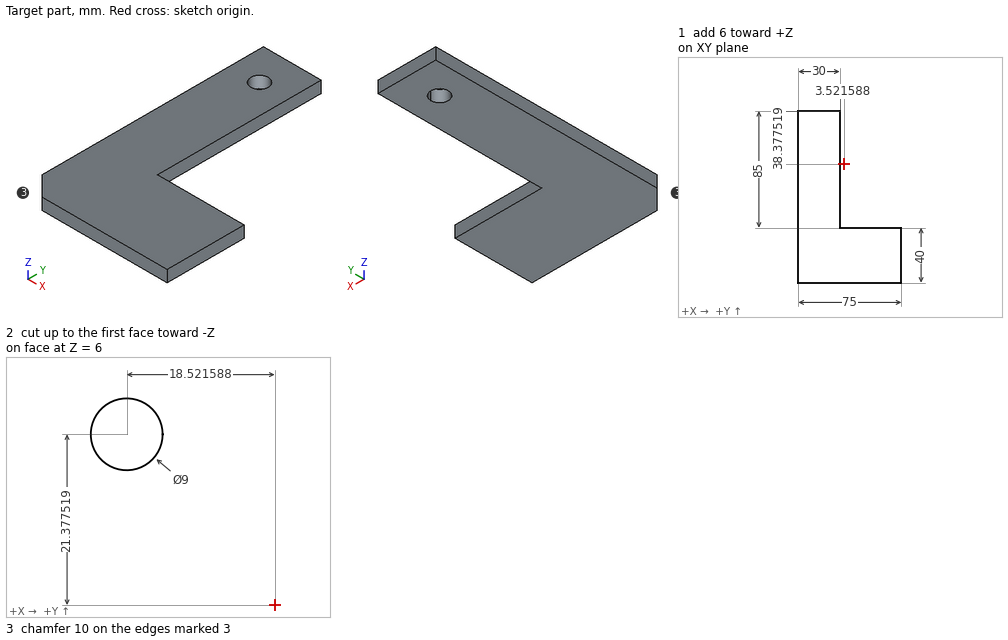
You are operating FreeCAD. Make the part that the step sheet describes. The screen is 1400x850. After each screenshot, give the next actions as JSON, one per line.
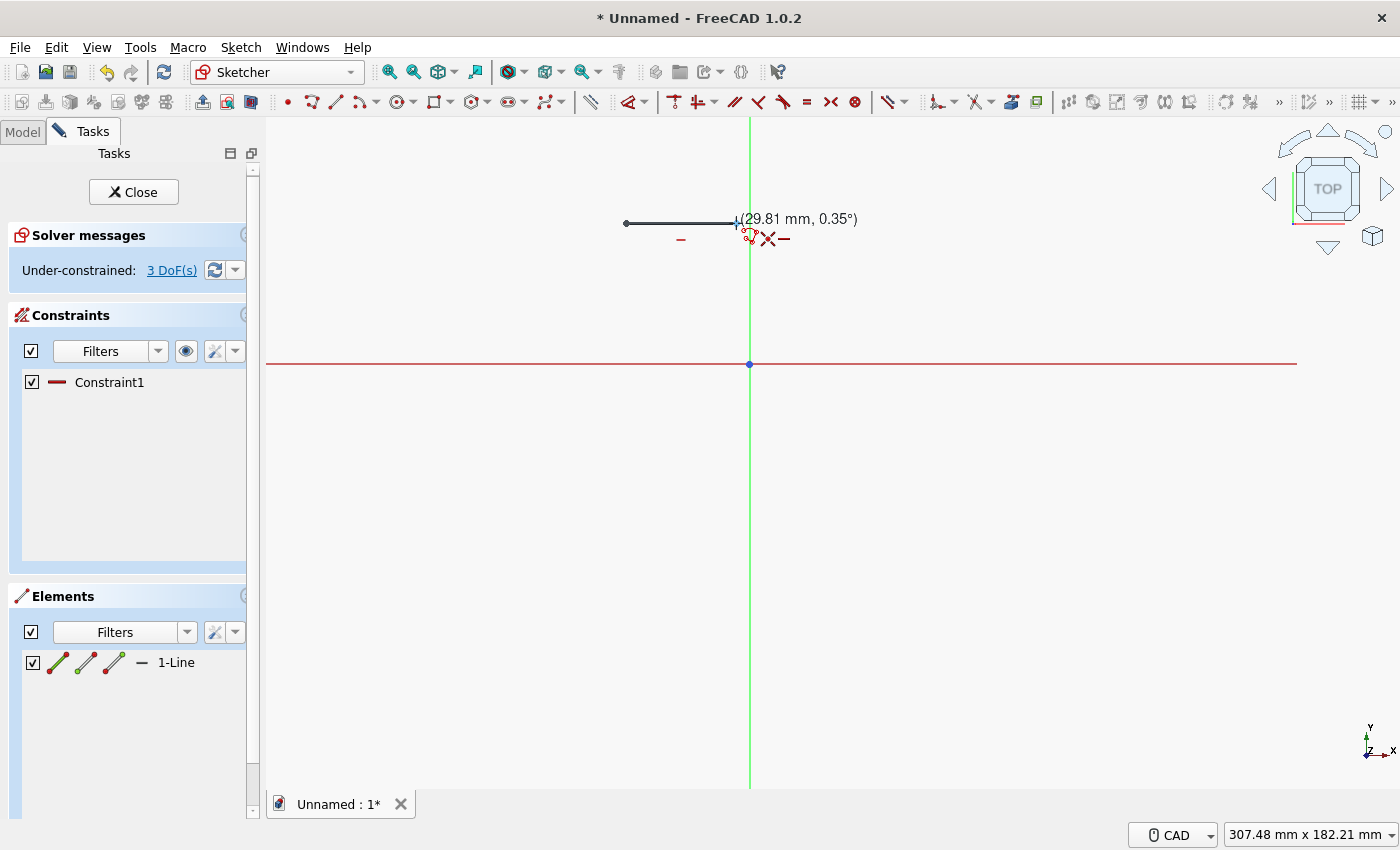
{"action": "left_click", "coordinate": [626, 684]}
{"action": "left_click", "coordinate": [903, 684]}
{"action": "left_click", "coordinate": [903, 536]}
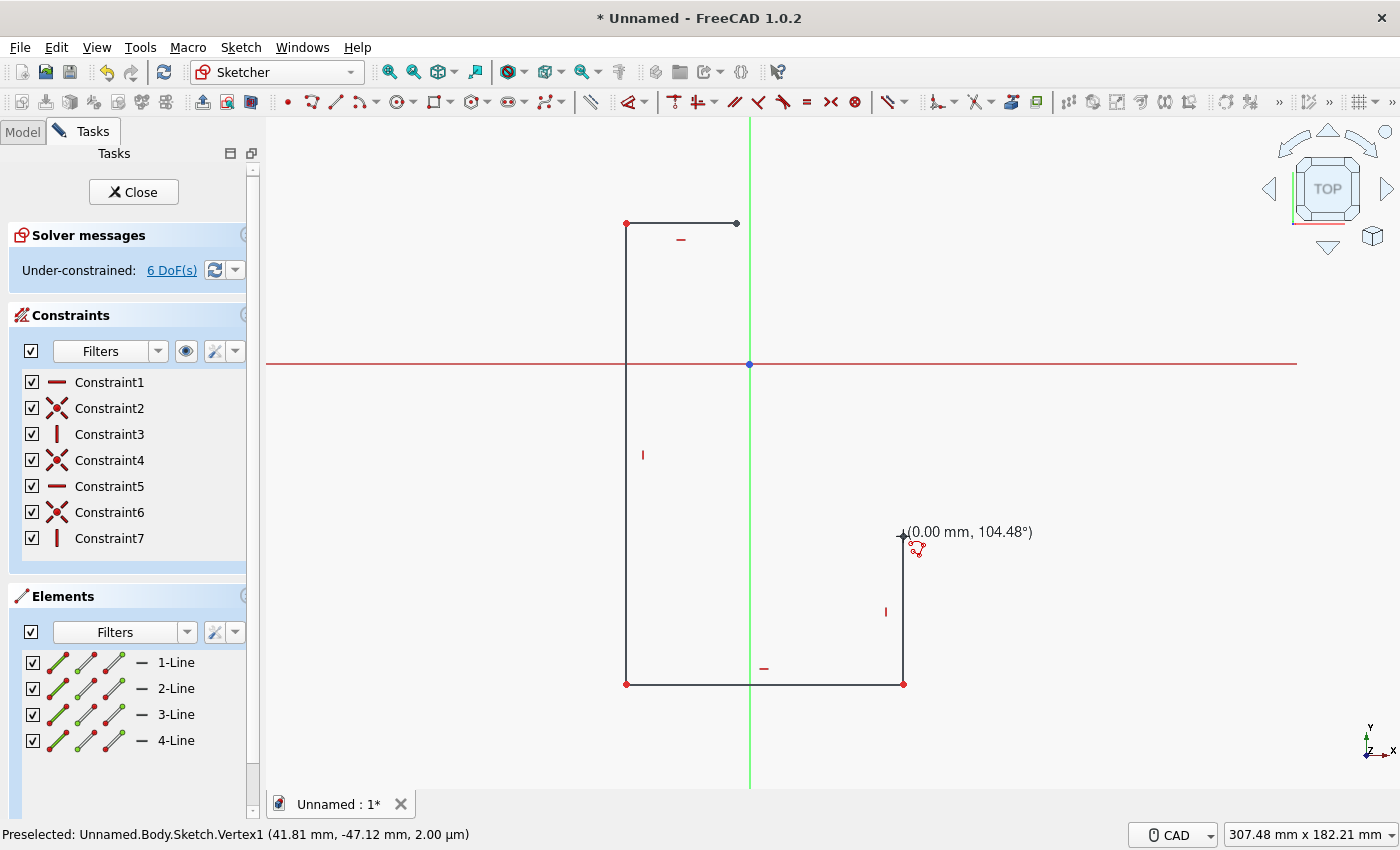
{"action": "scroll", "coordinate": [737, 536], "scroll_direction": "up", "scroll_amount": 2}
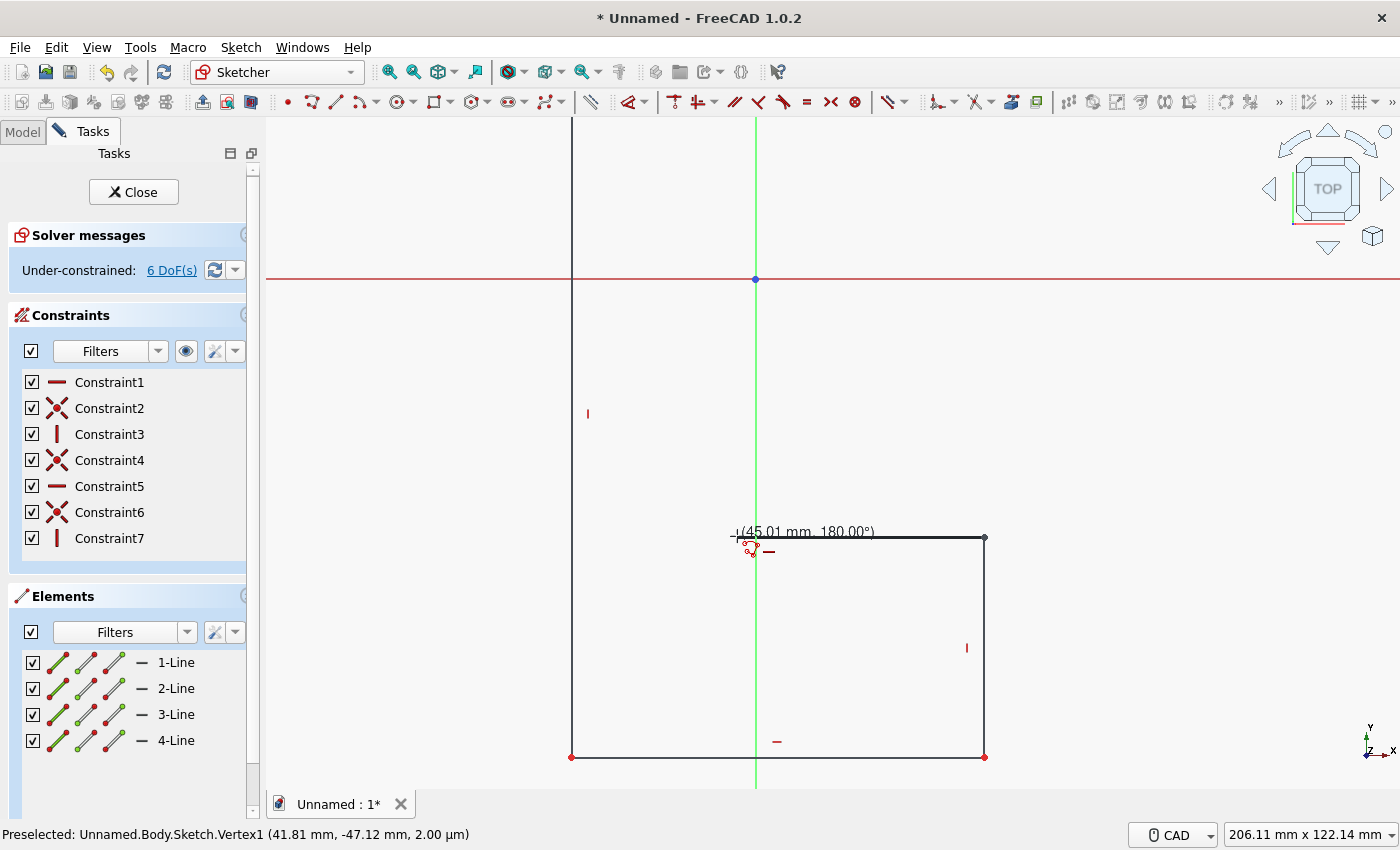
{"action": "left_click", "coordinate": [737, 536]}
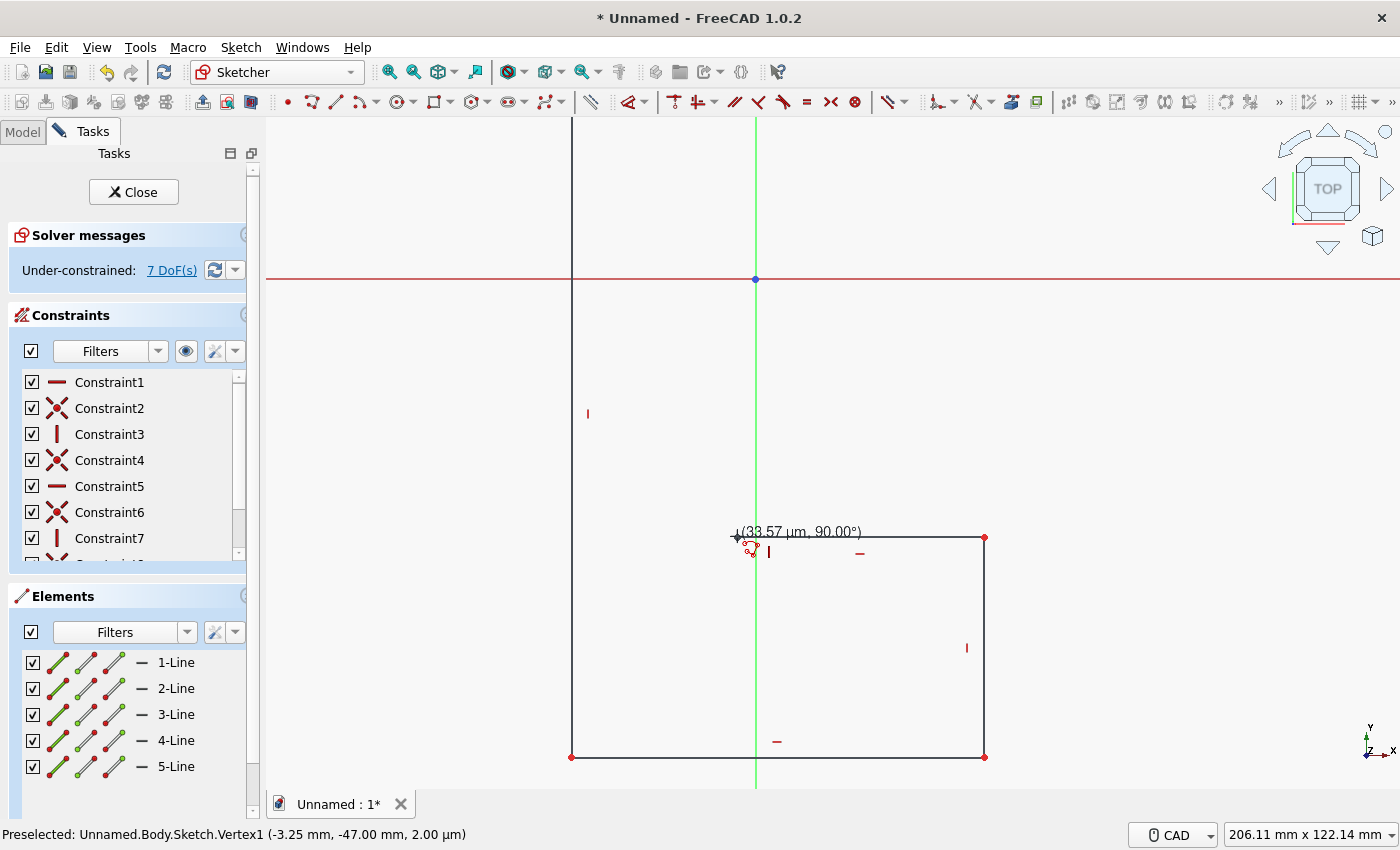
{"action": "scroll", "coordinate": [737, 536], "scroll_direction": "down", "scroll_amount": 2}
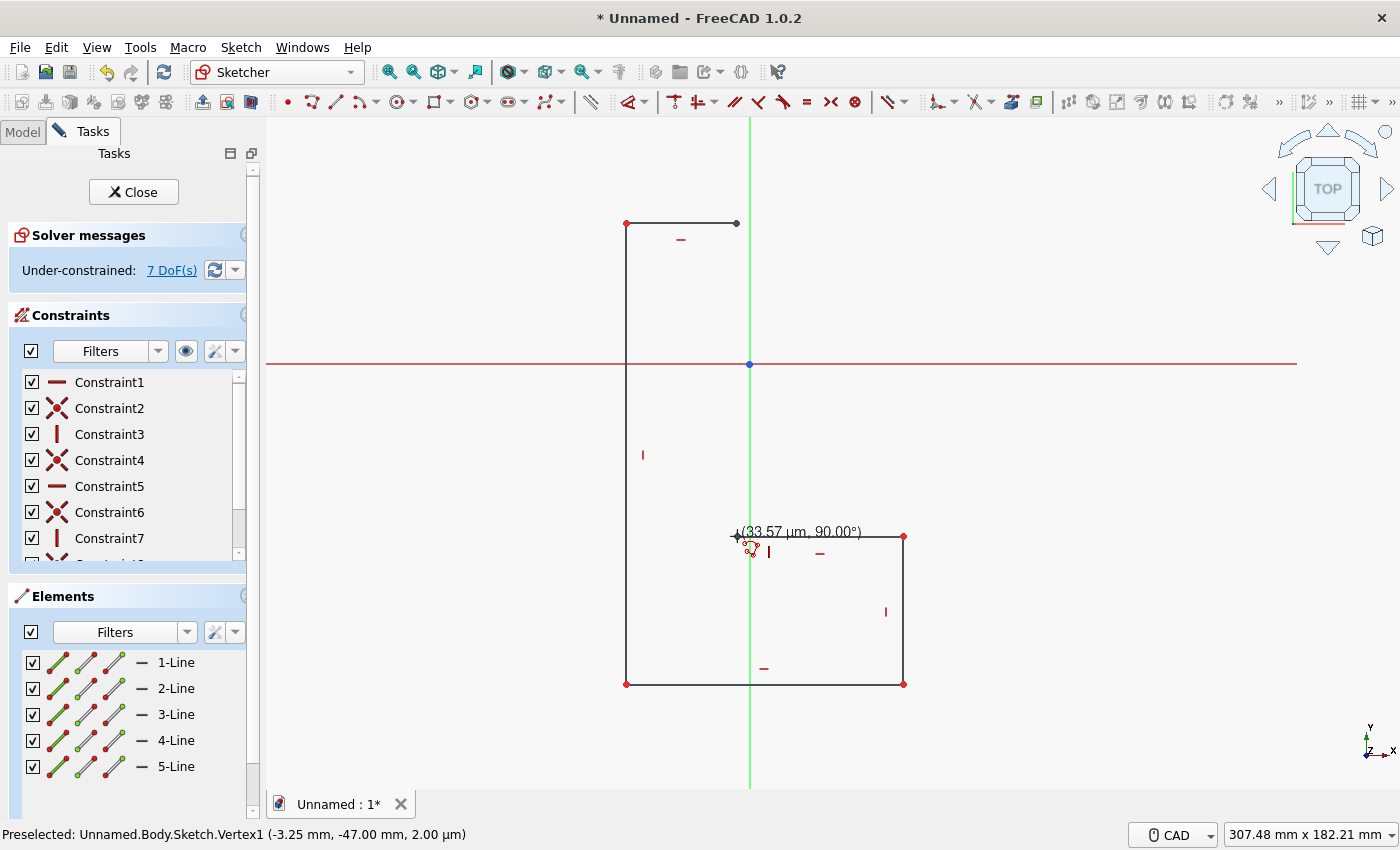
{"action": "scroll", "coordinate": [737, 223], "scroll_direction": "up", "scroll_amount": 2}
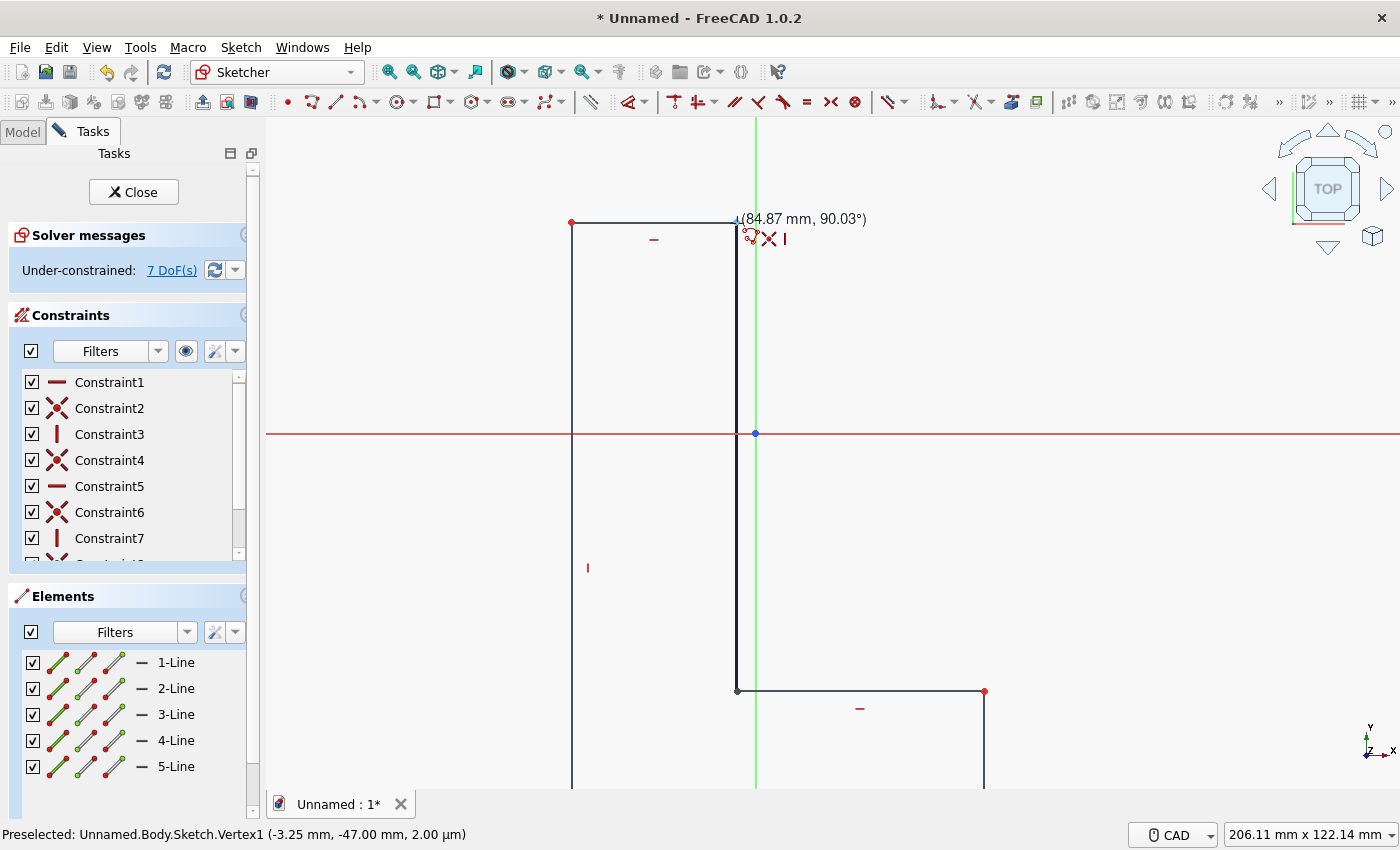
{"action": "left_click", "coordinate": [737, 223]}
{"action": "key", "text": "Escape"}
{"action": "key", "text": "Escape"}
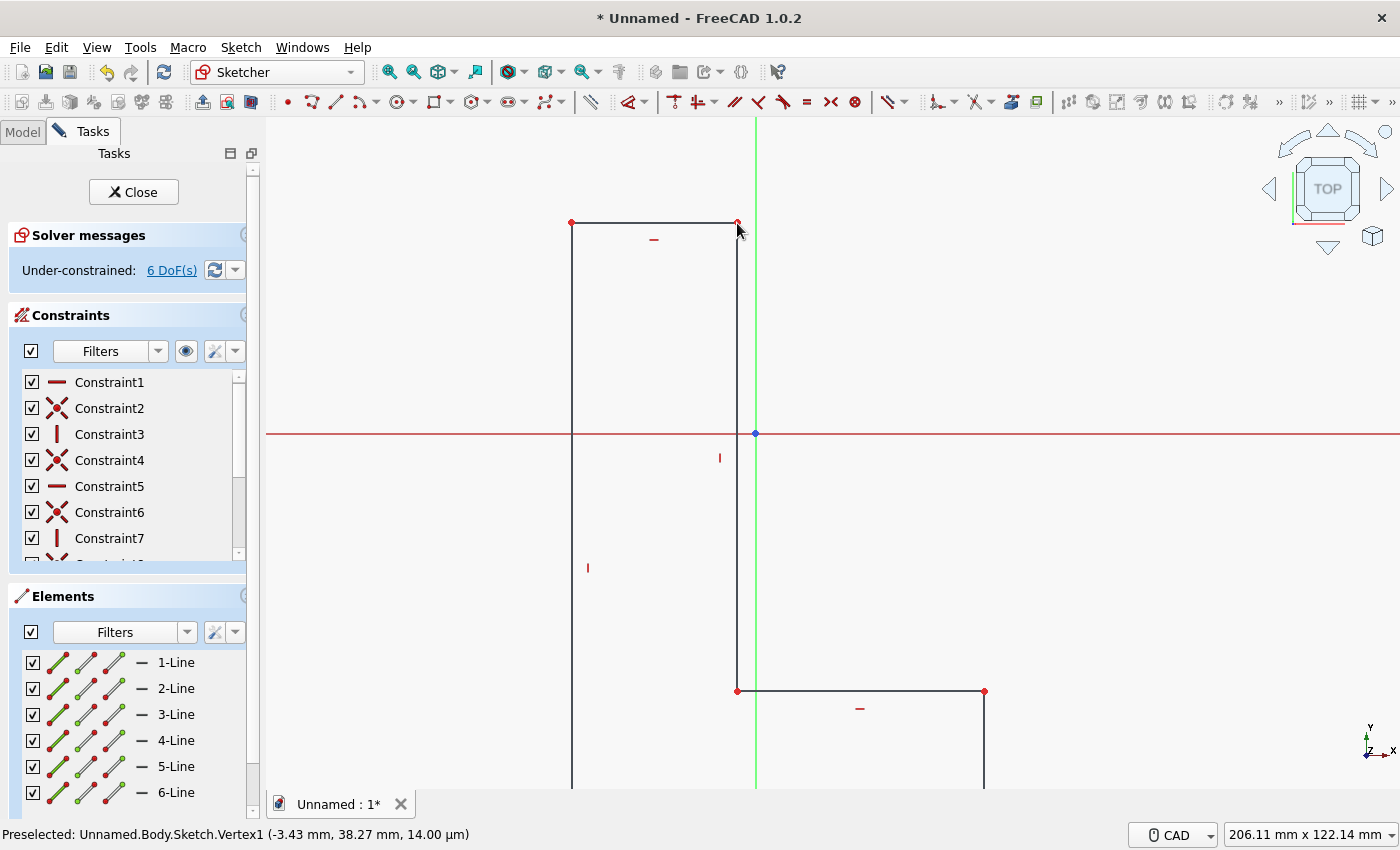
{"action": "left_click", "coordinate": [687, 223]}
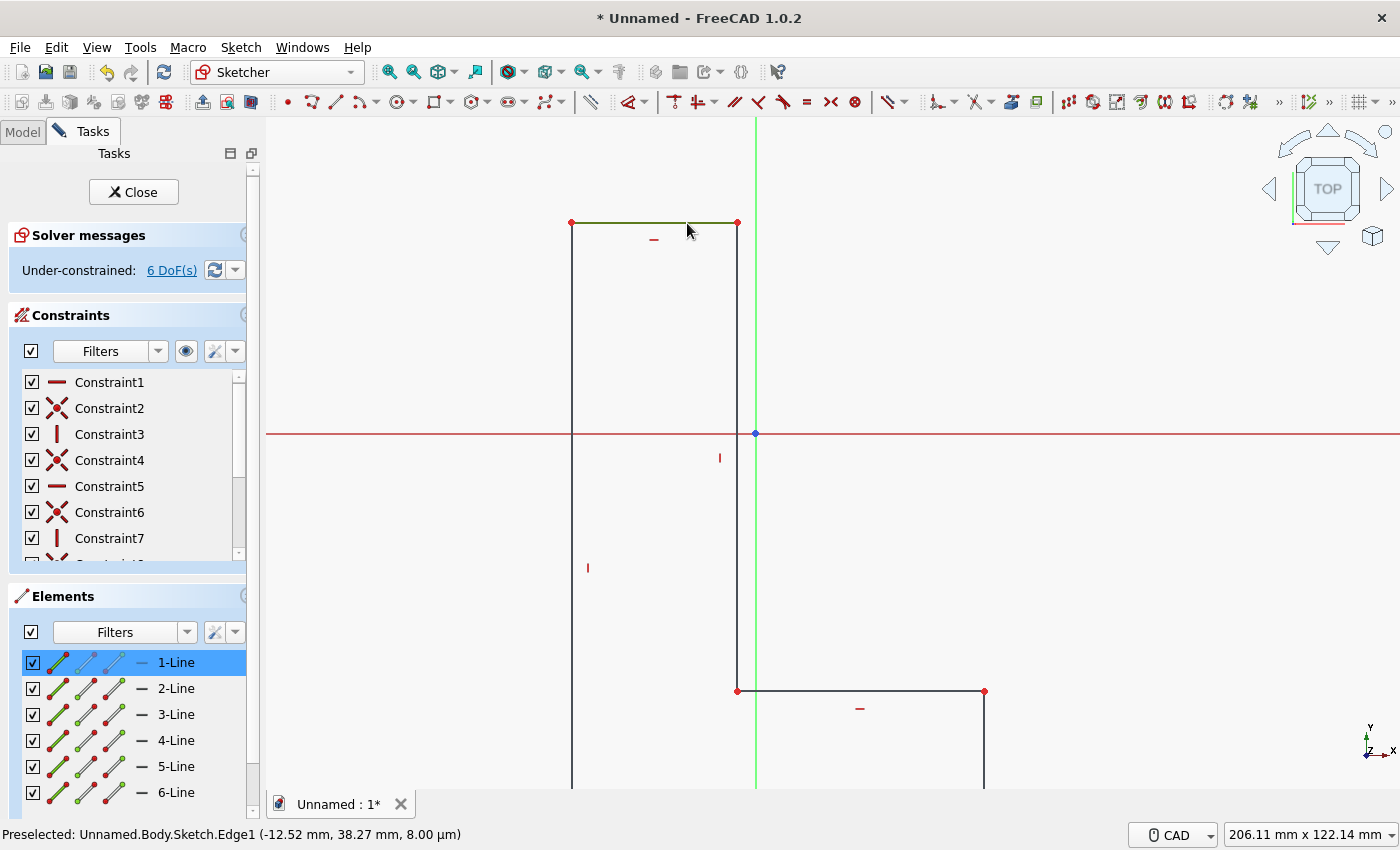
{"action": "key", "text": "l"}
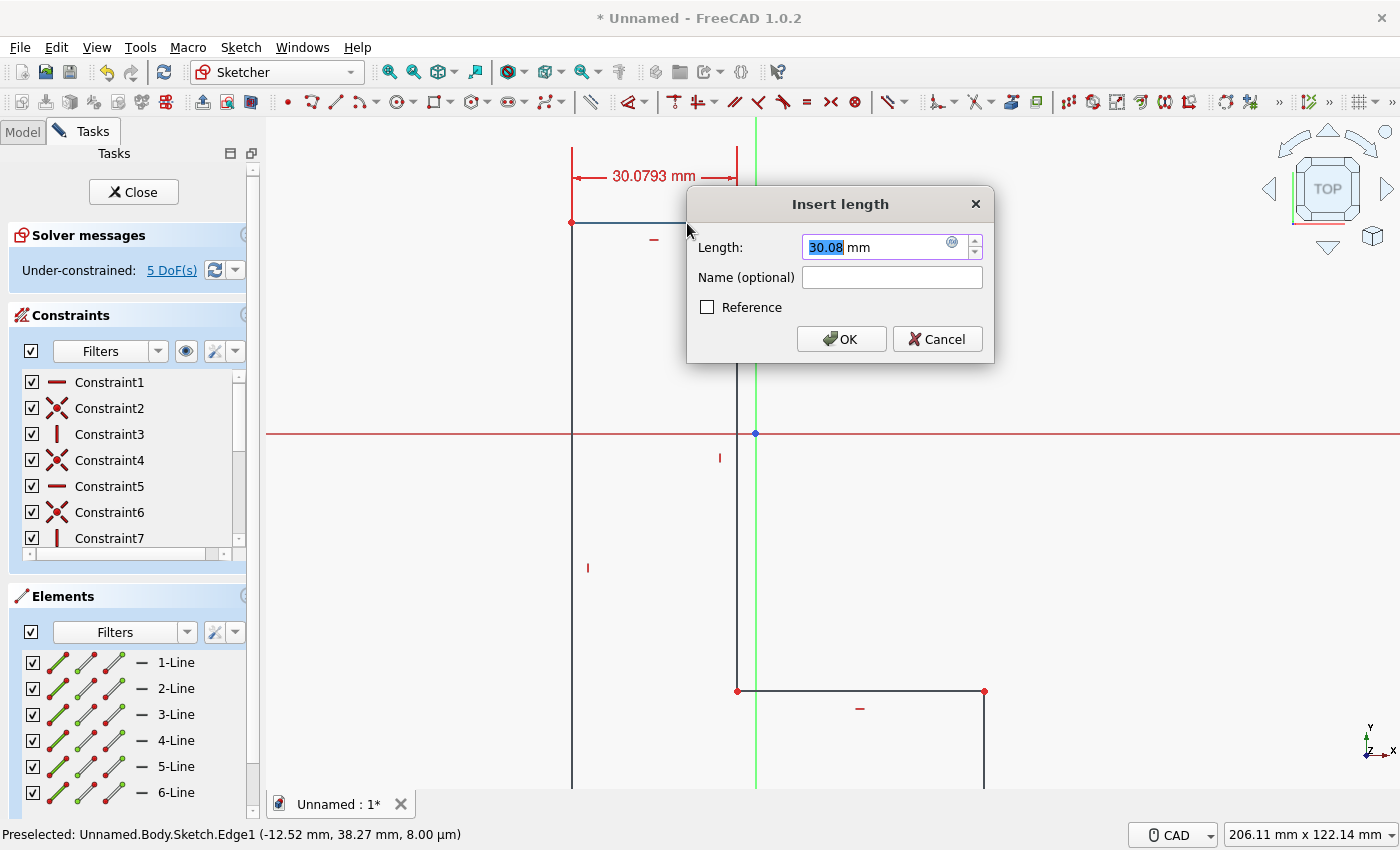
{"action": "type", "text": "30"}
{"action": "key", "text": "Return"}